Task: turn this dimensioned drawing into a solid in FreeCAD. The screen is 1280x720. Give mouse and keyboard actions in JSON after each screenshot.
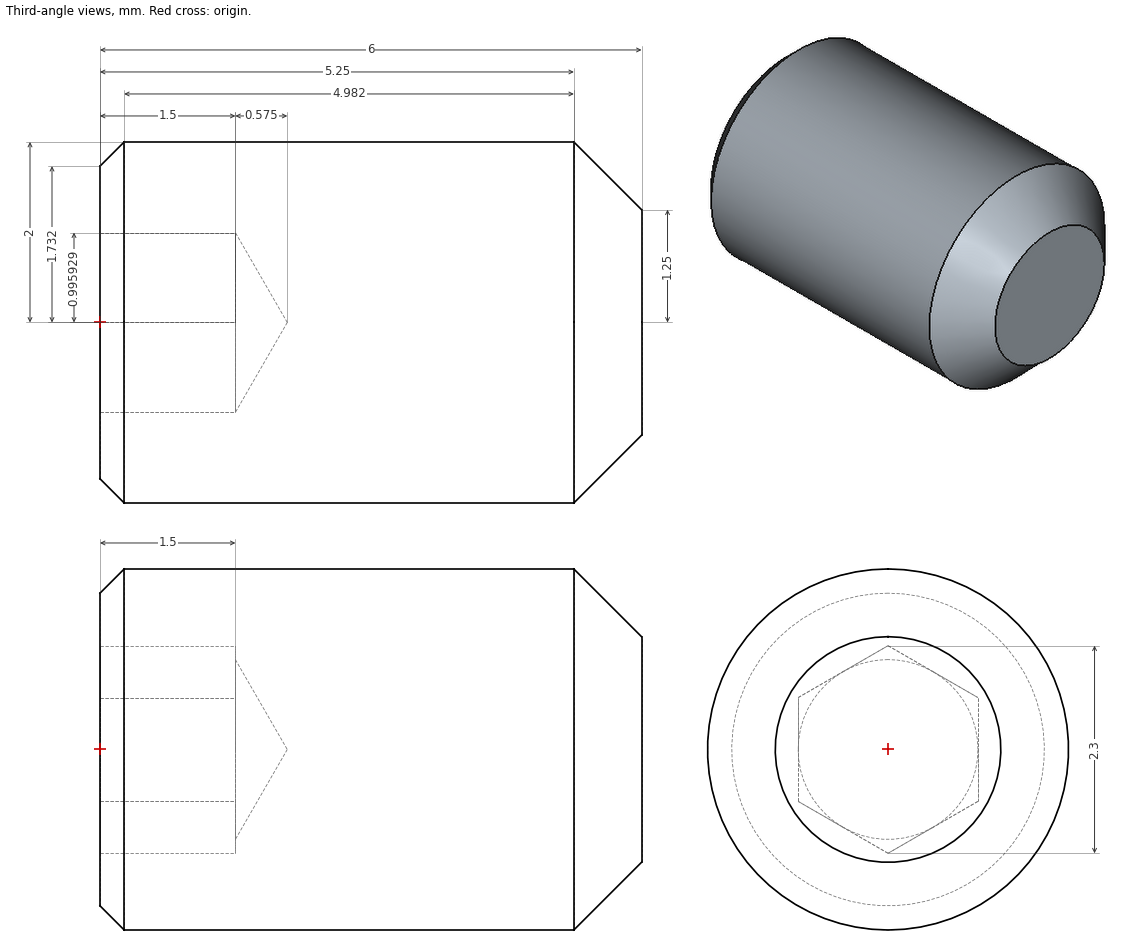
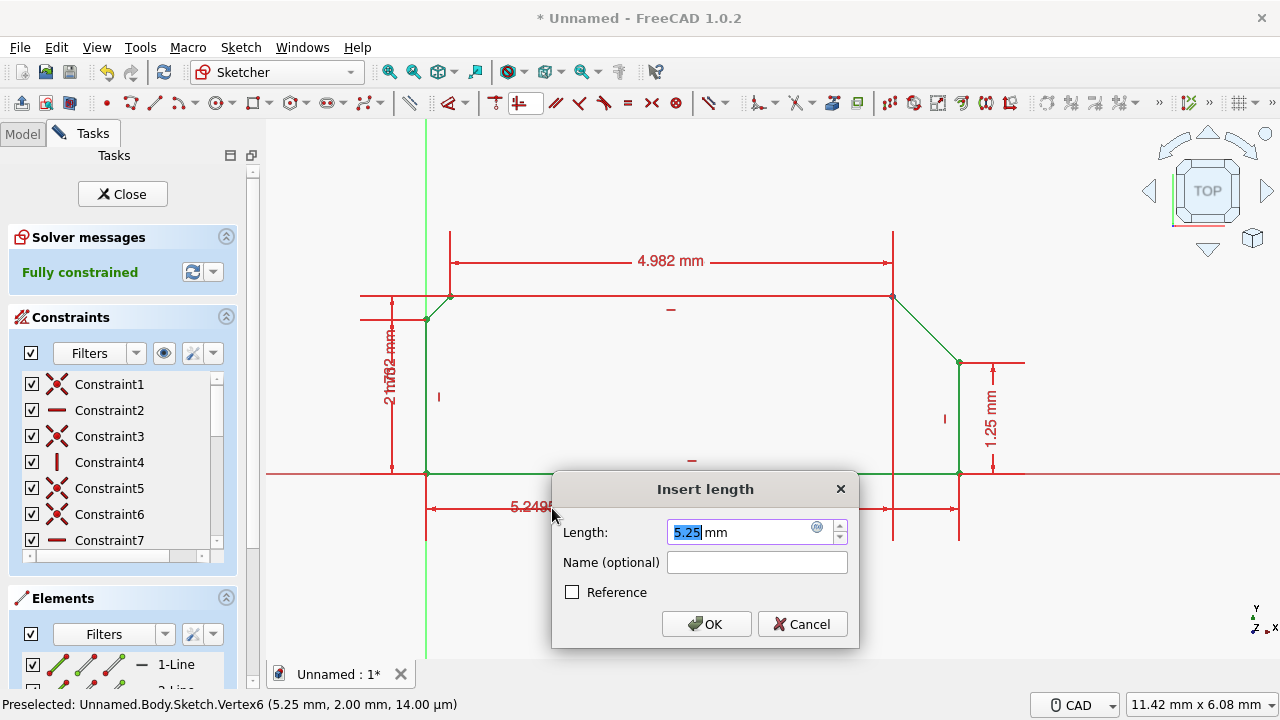
{"action": "type", "text": "5.25"}
{"action": "key", "text": "Return"}
{"action": "key", "text": "Escape"}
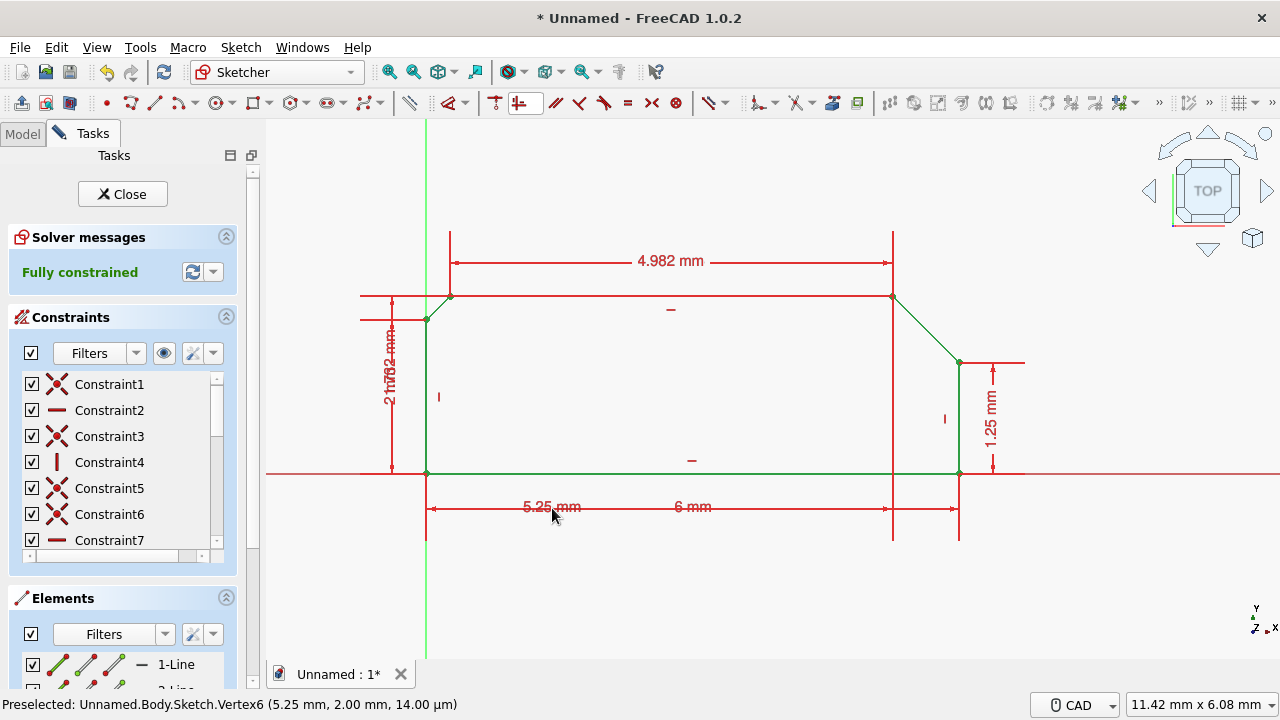
{"action": "left_click", "coordinate": [123, 194]}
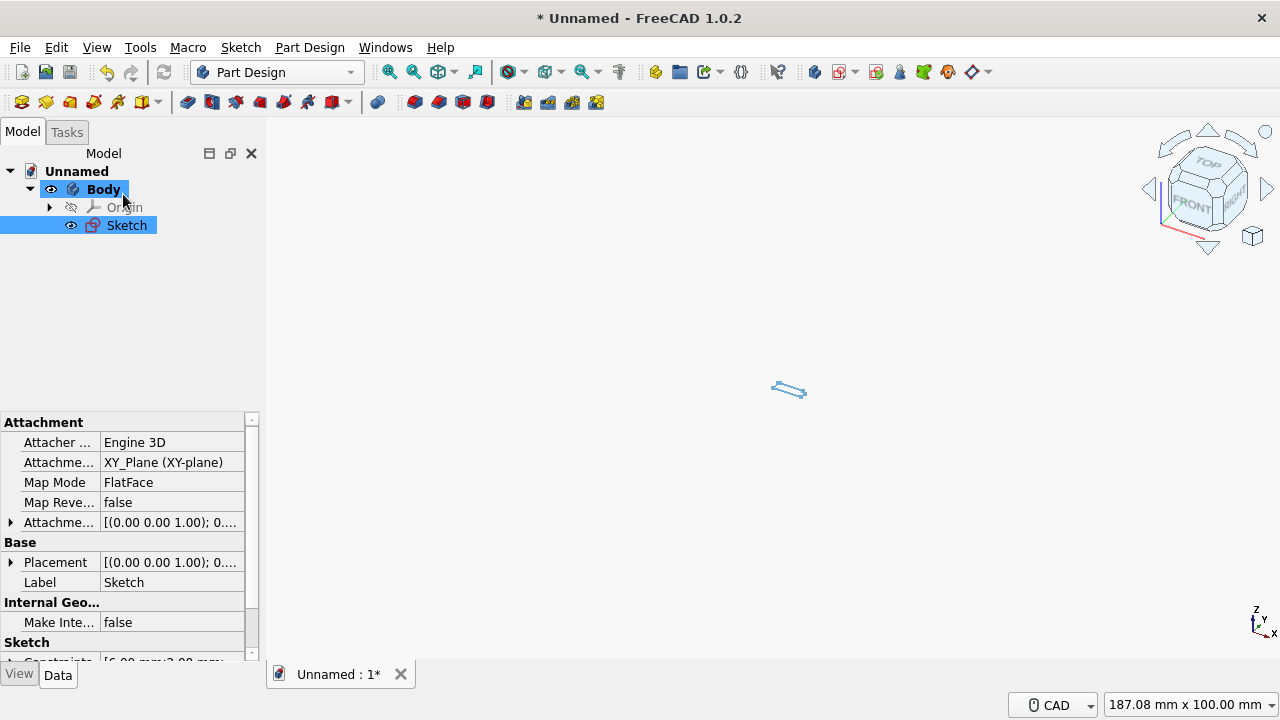
{"action": "left_click", "coordinate": [46, 102]}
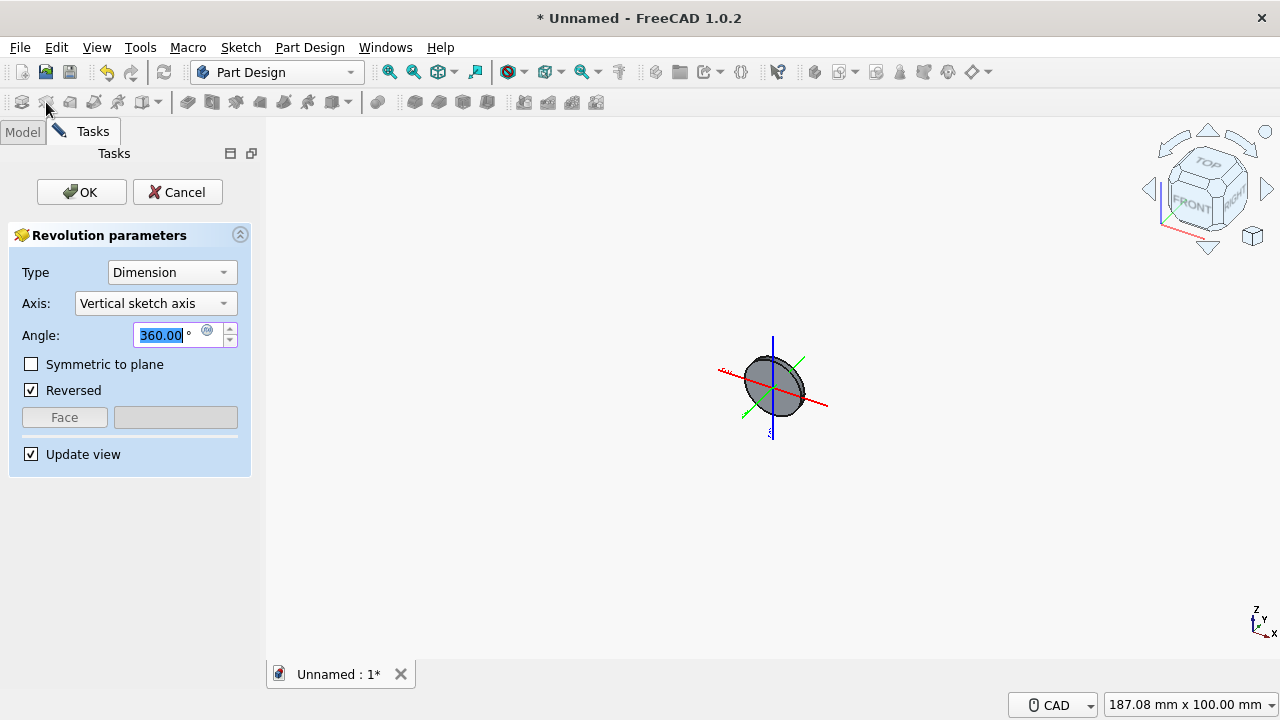
{"action": "left_click", "coordinate": [156, 304]}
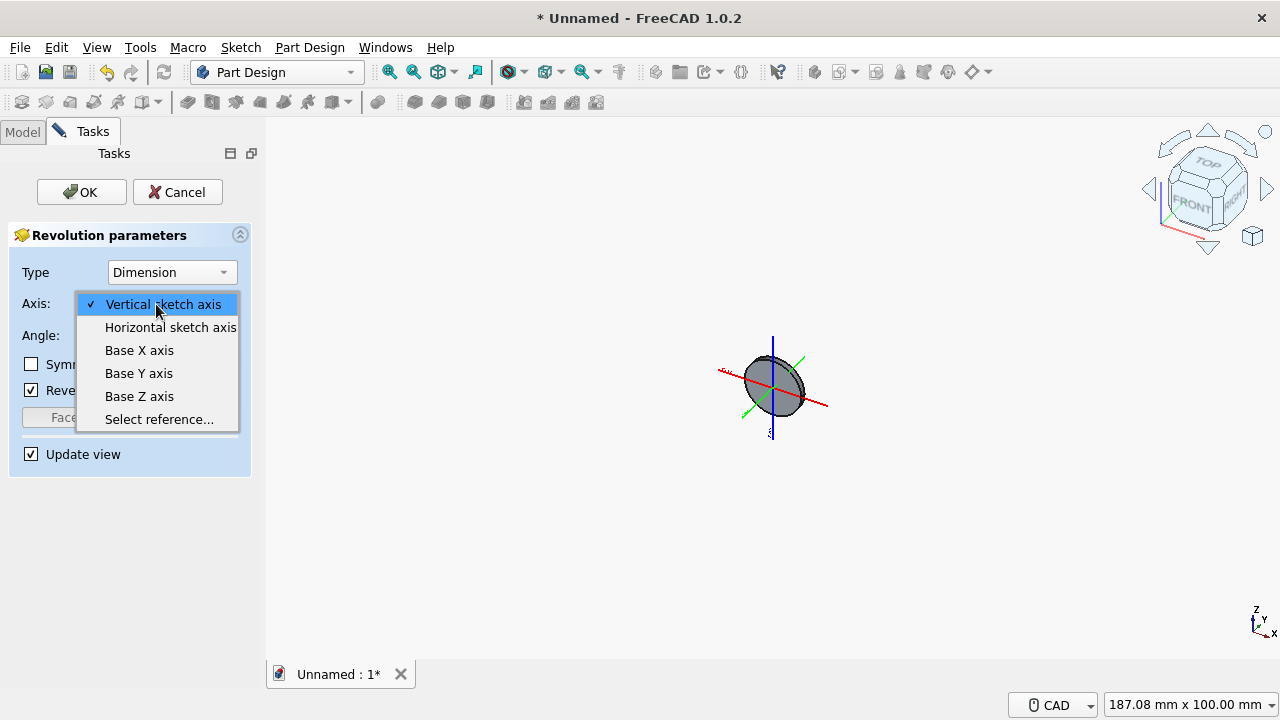
{"action": "left_click", "coordinate": [156, 328]}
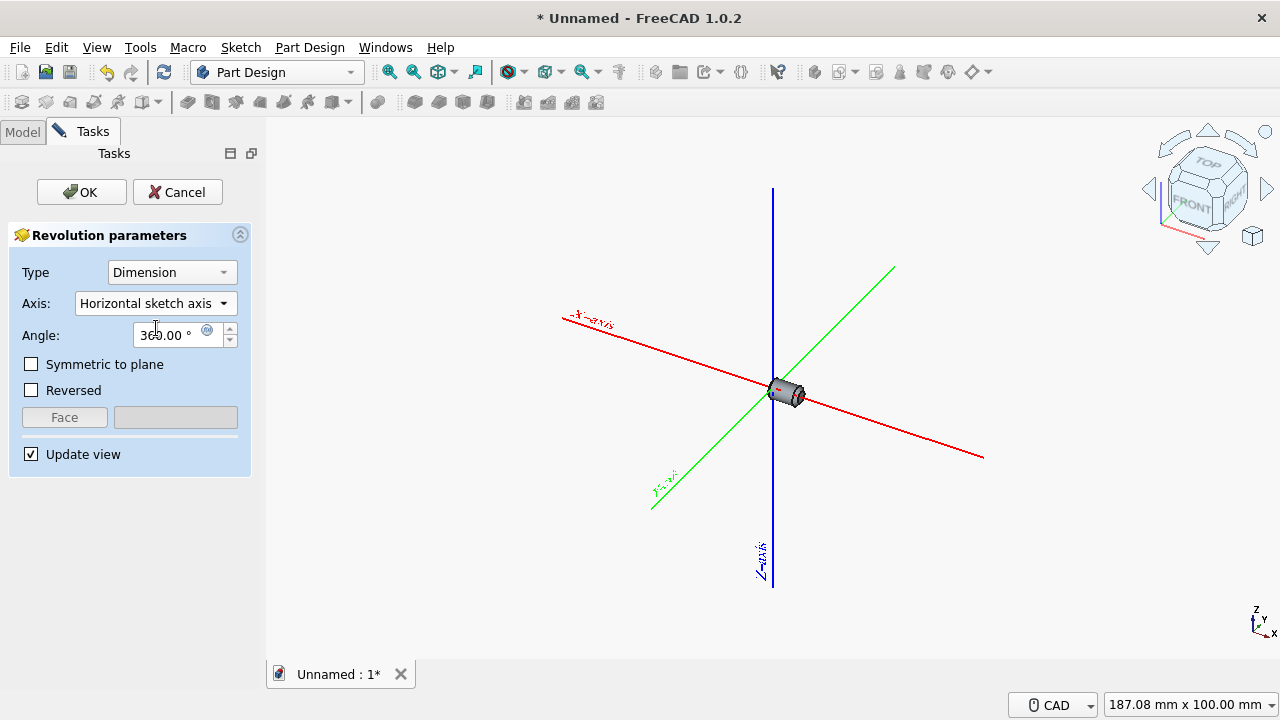
{"action": "left_click", "coordinate": [82, 192]}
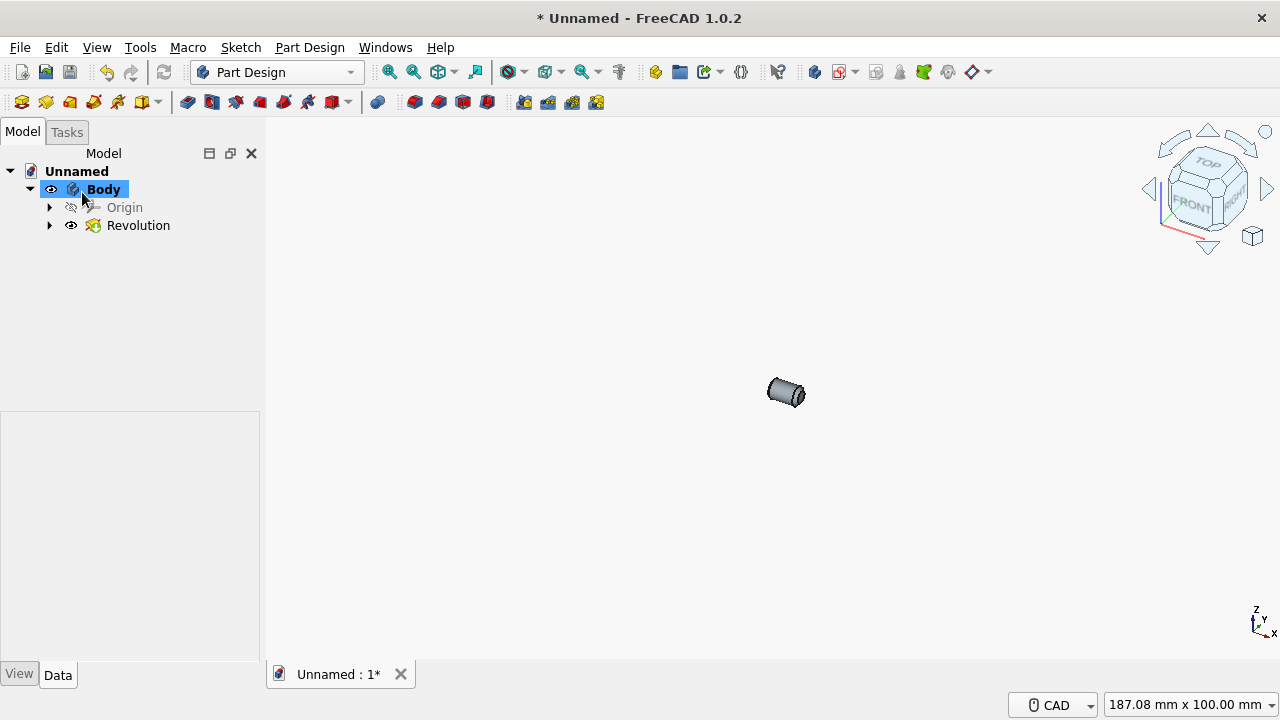
{"action": "left_click", "coordinate": [390, 72]}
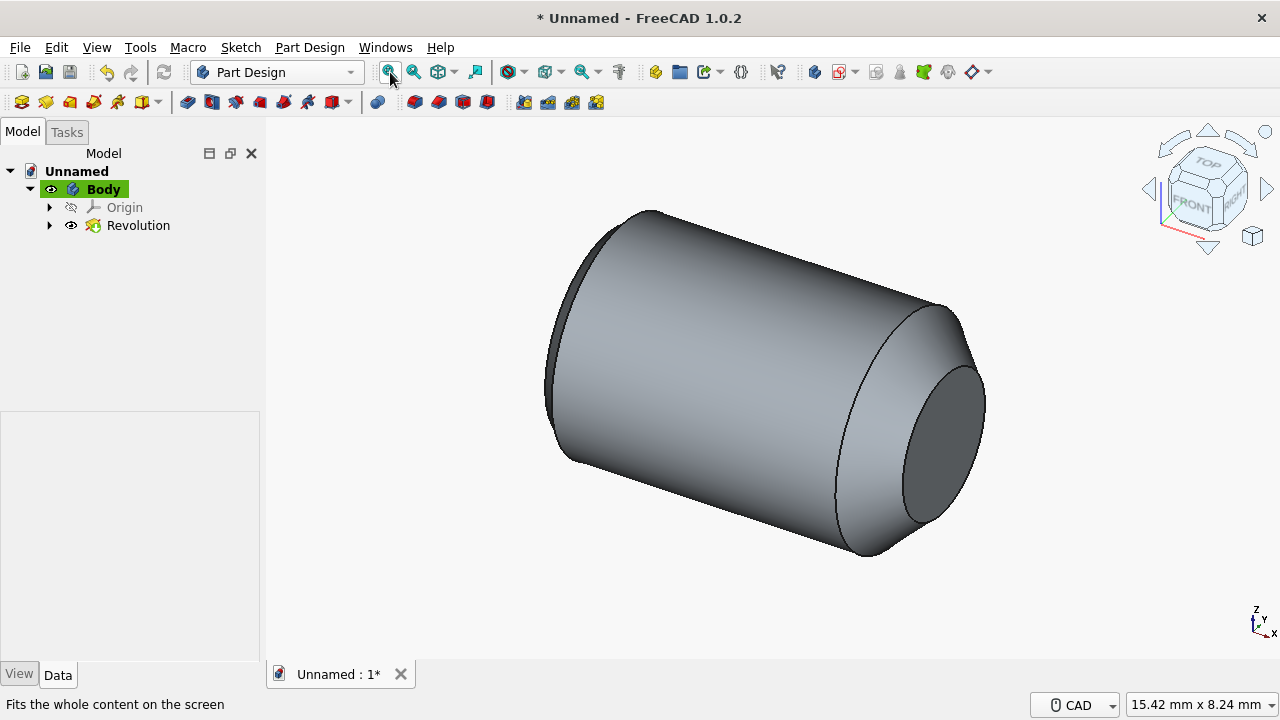
{"action": "key", "text": "6"}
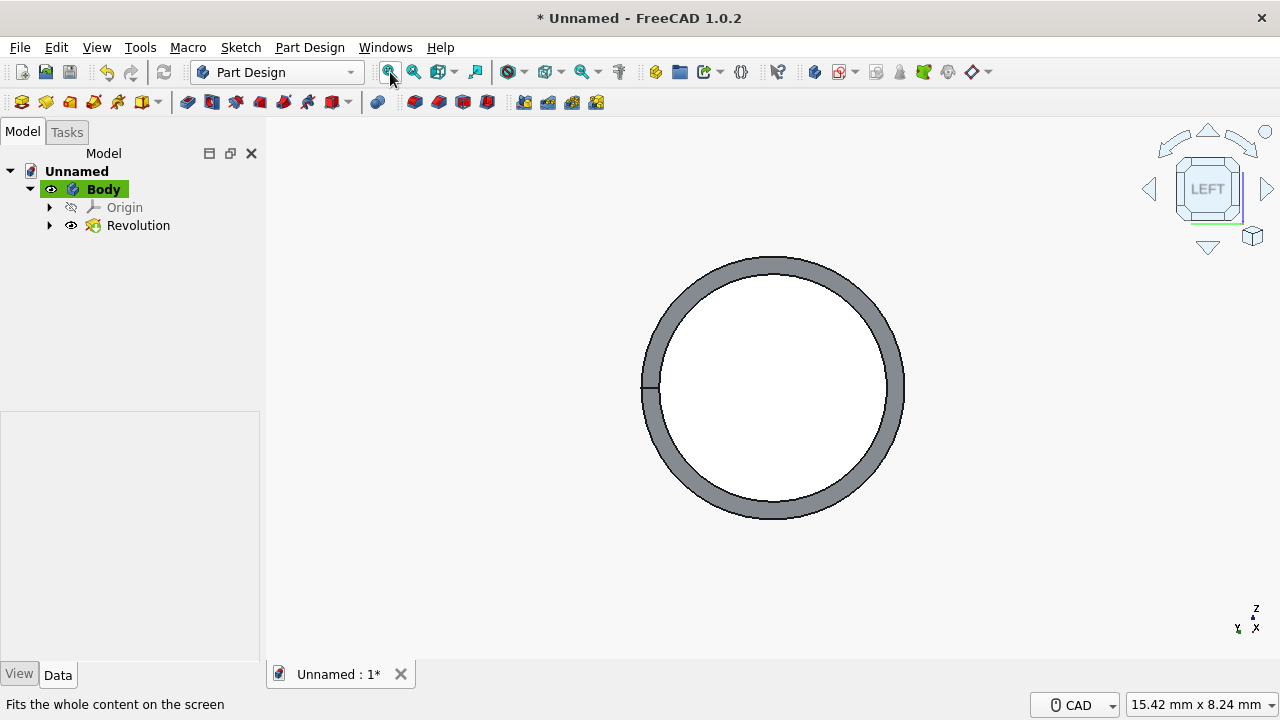
{"action": "left_click", "coordinate": [773, 387]}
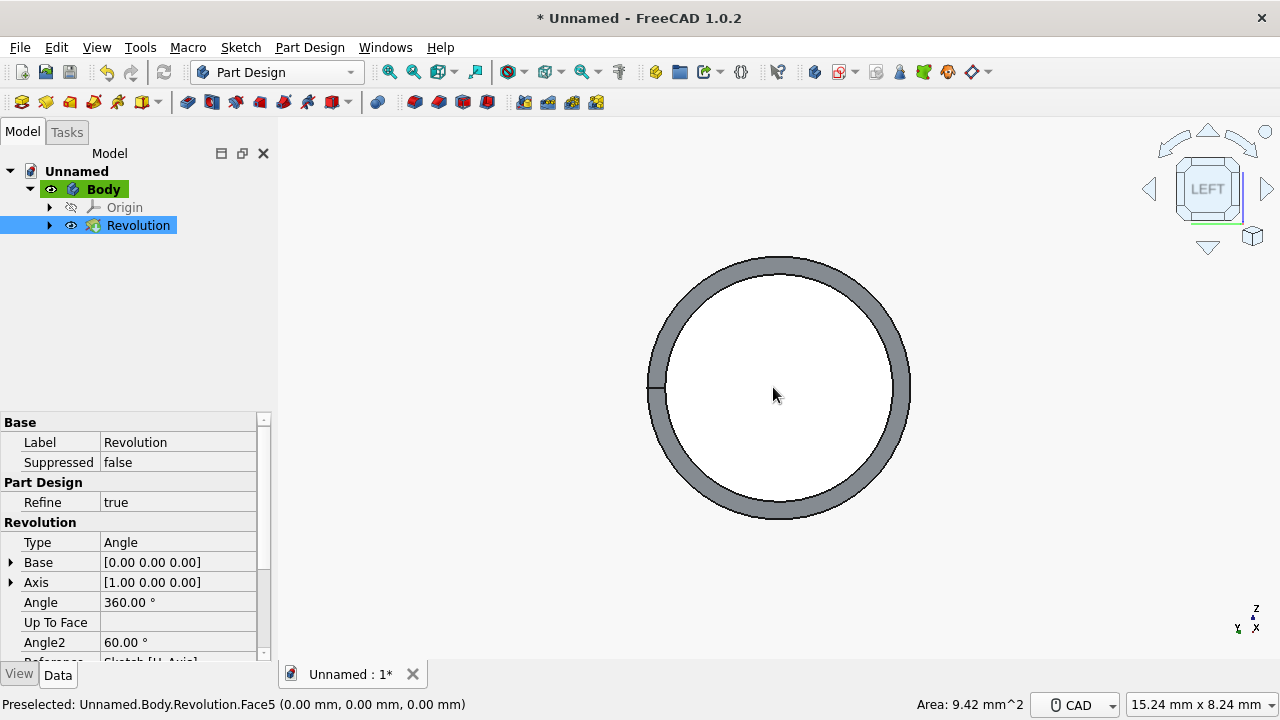
{"action": "left_click", "coordinate": [840, 72]}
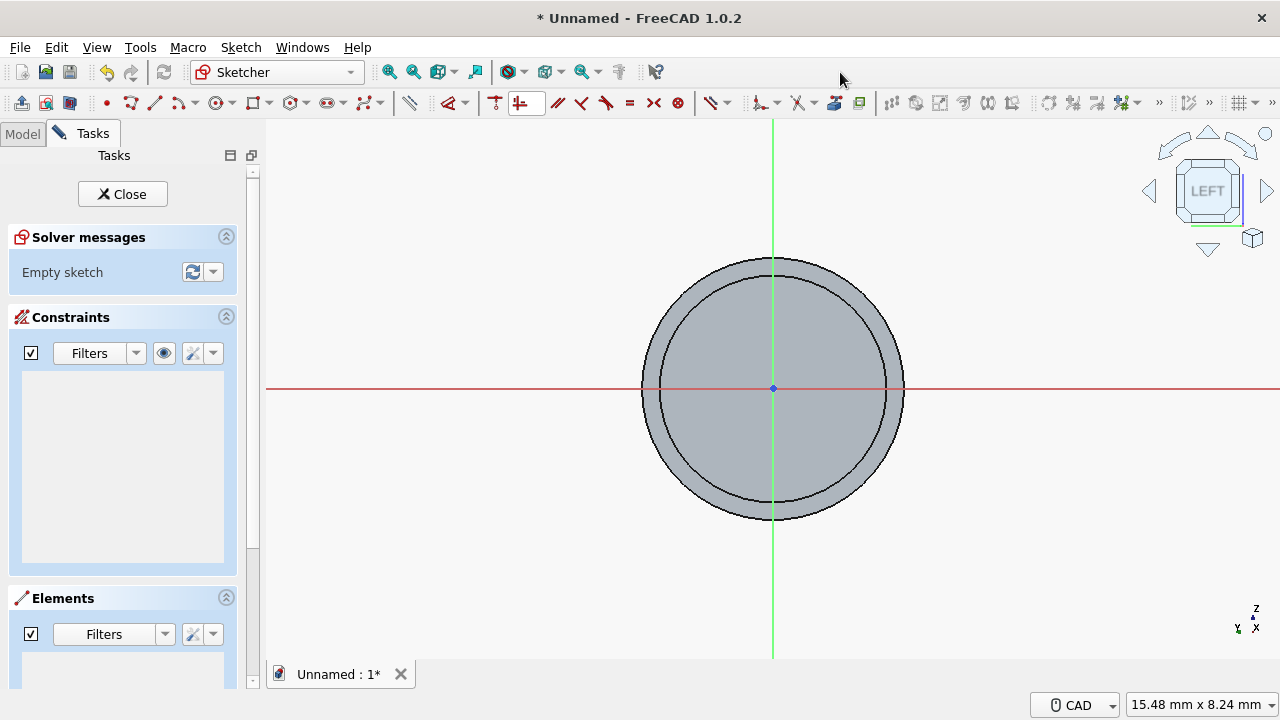
{"action": "scroll", "coordinate": [829, 389], "scroll_direction": "up", "scroll_amount": 4}